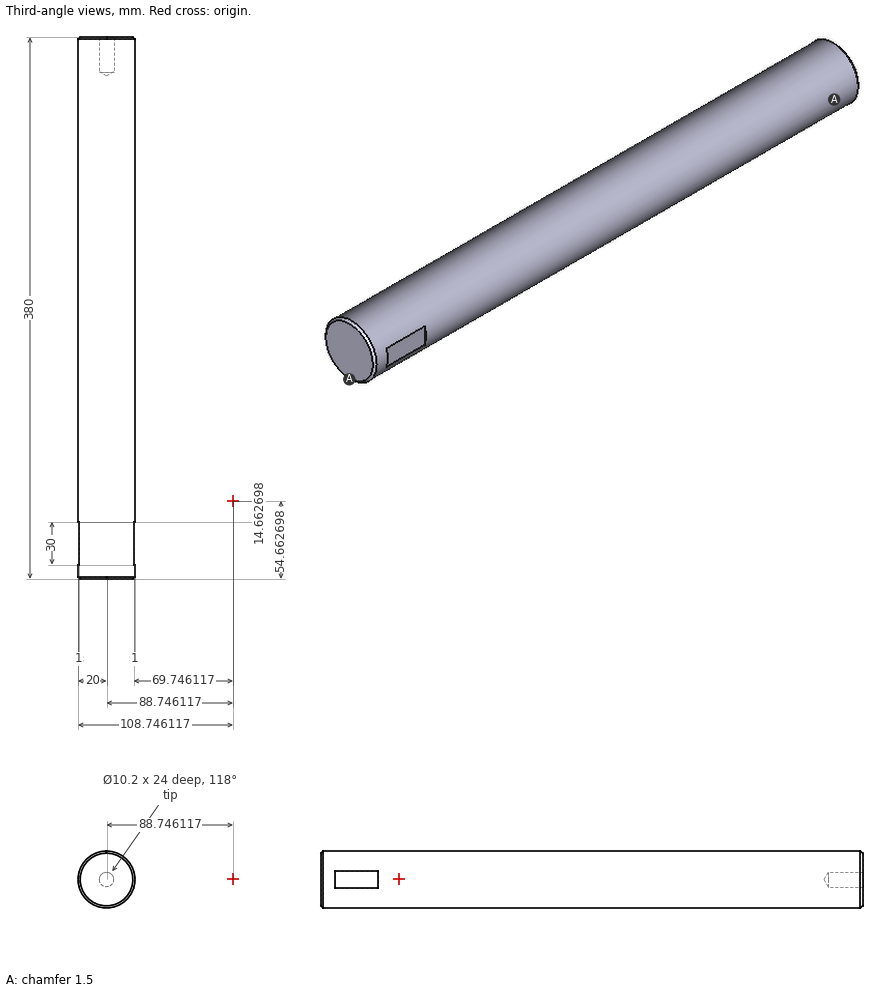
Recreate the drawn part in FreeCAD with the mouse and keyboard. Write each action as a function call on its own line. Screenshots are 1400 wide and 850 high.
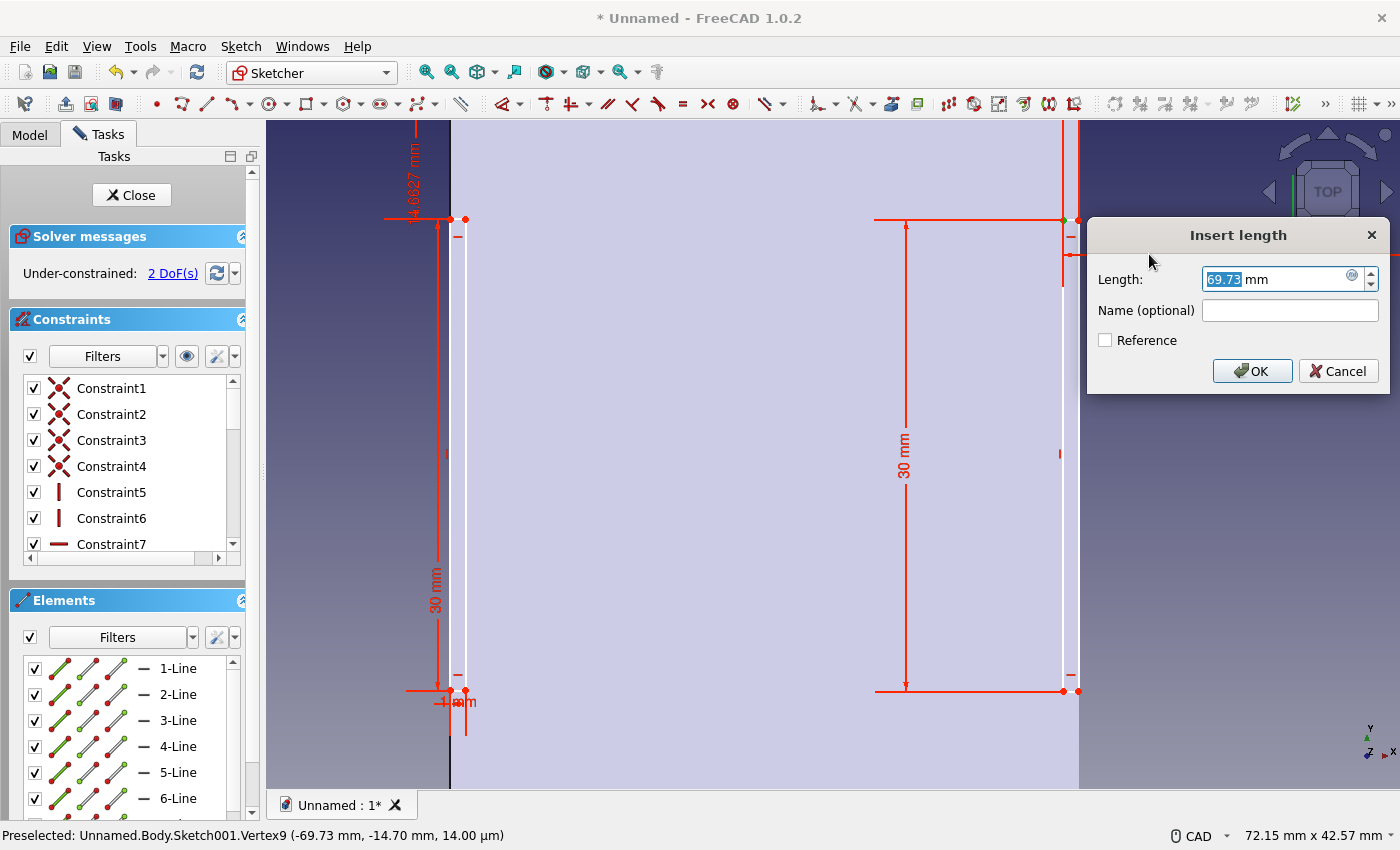
text(69.746117)
key(Return)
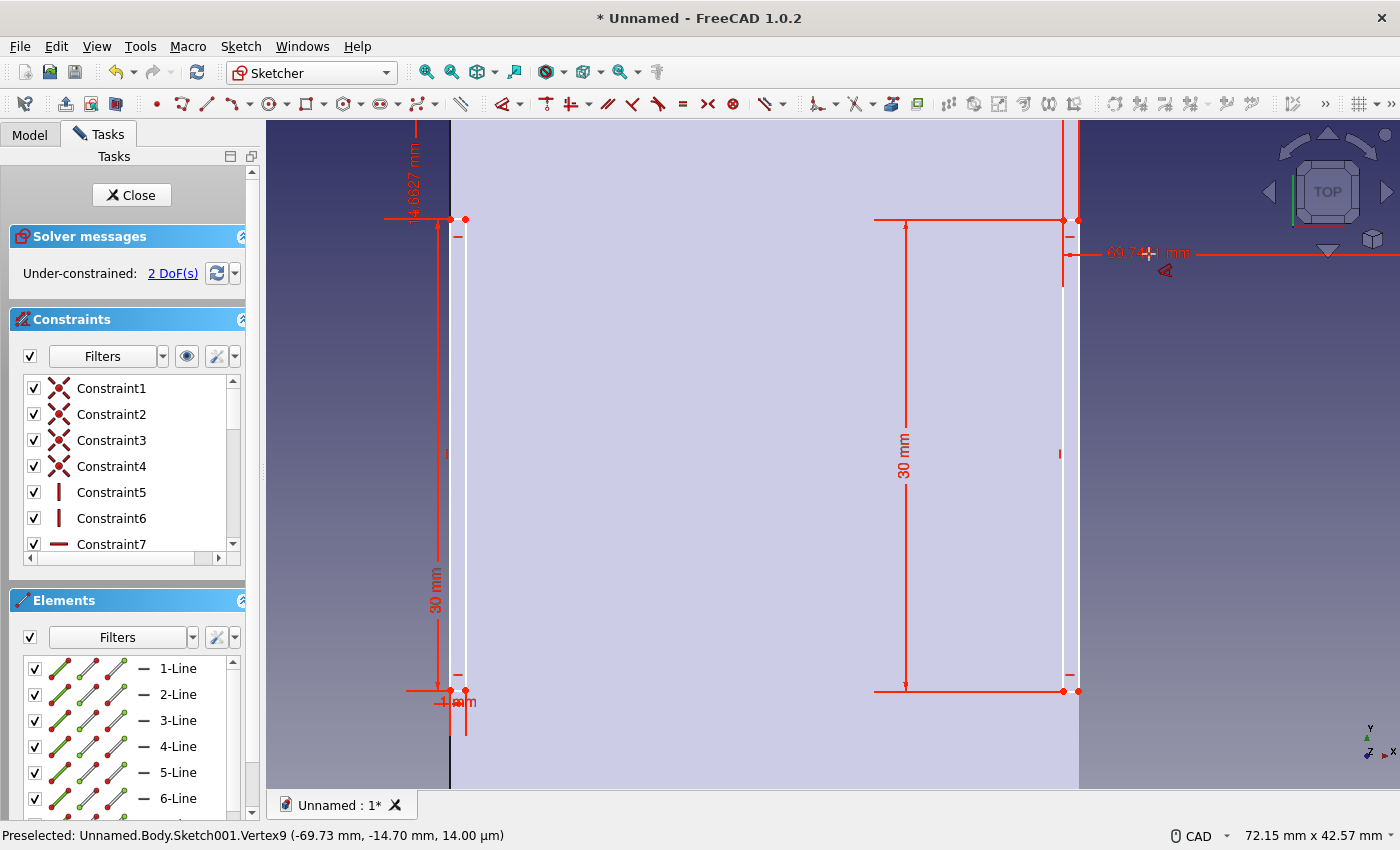
click(1063, 220)
click(1029, 184)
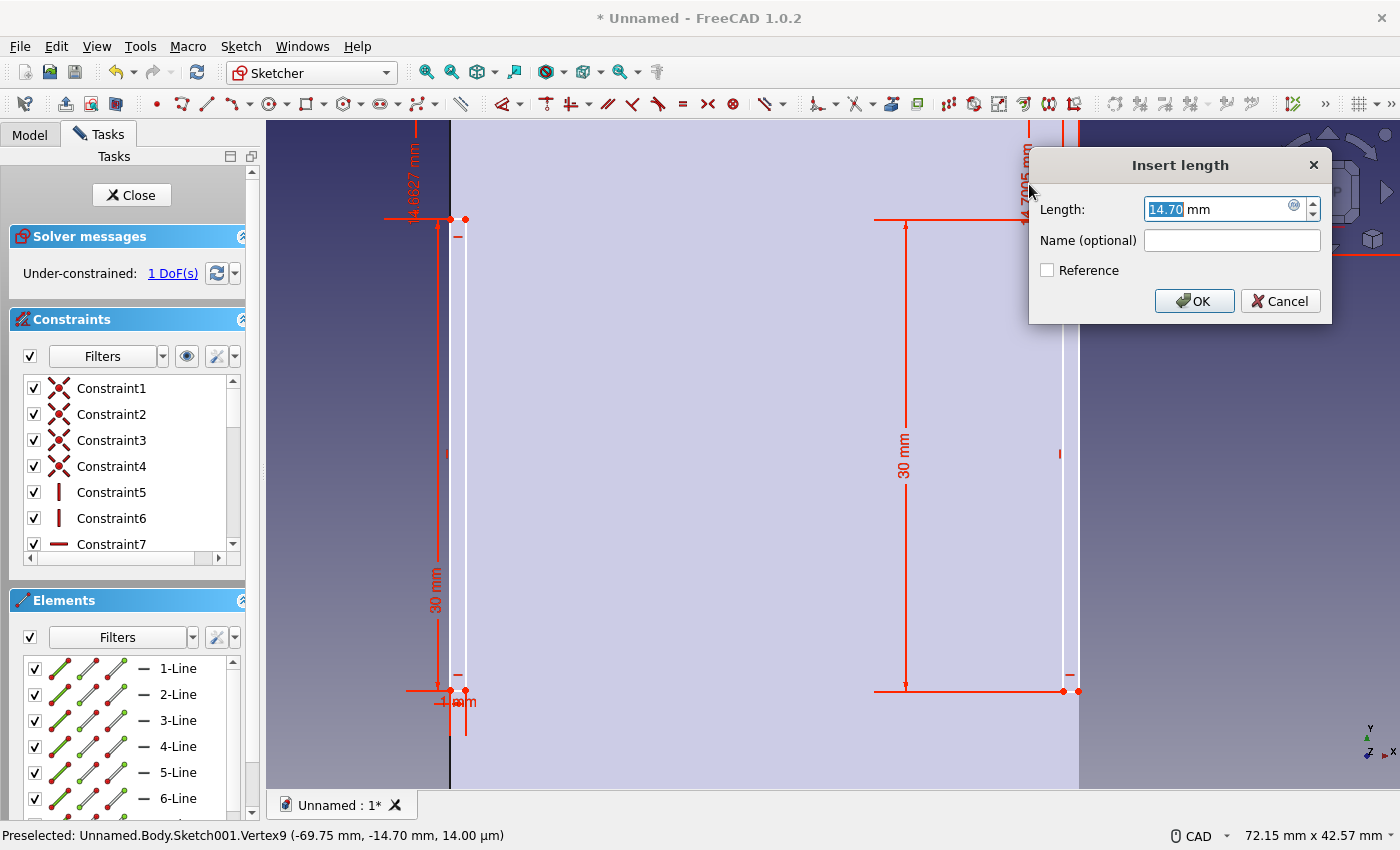
text(14.662698)
key(Return)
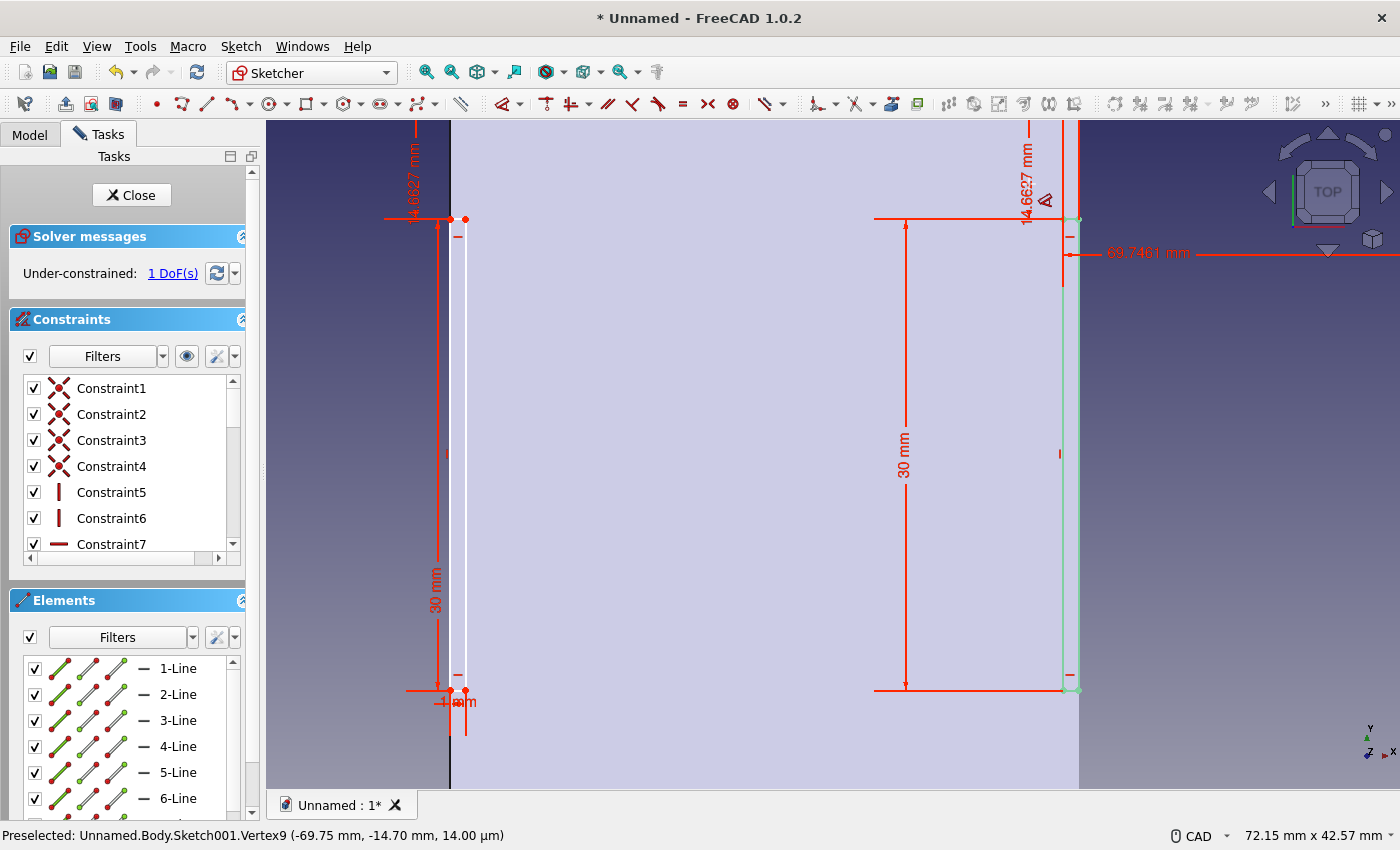
click(450, 219)
click(843, 253)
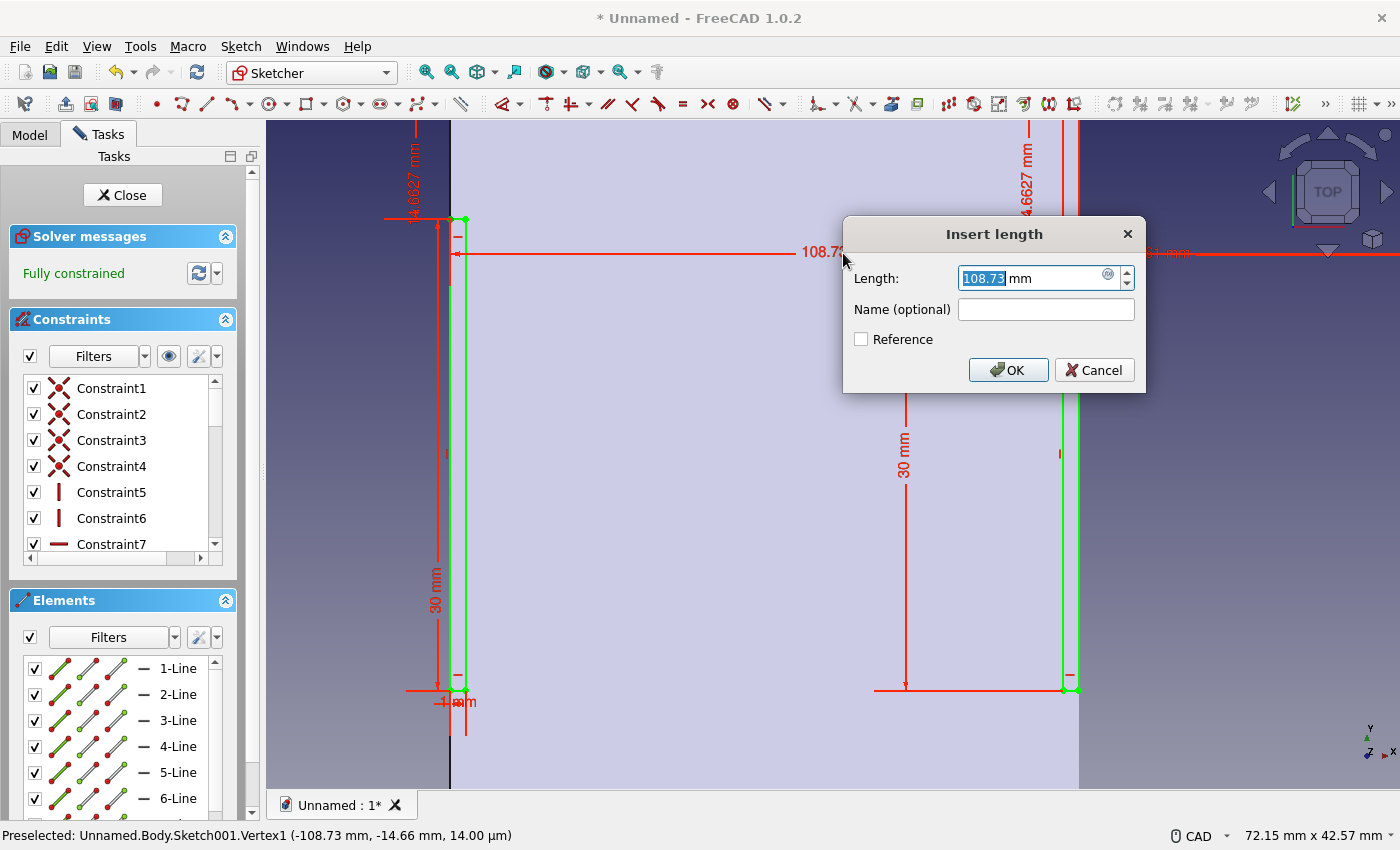
text(108.746117)
key(Return)
key(Escape)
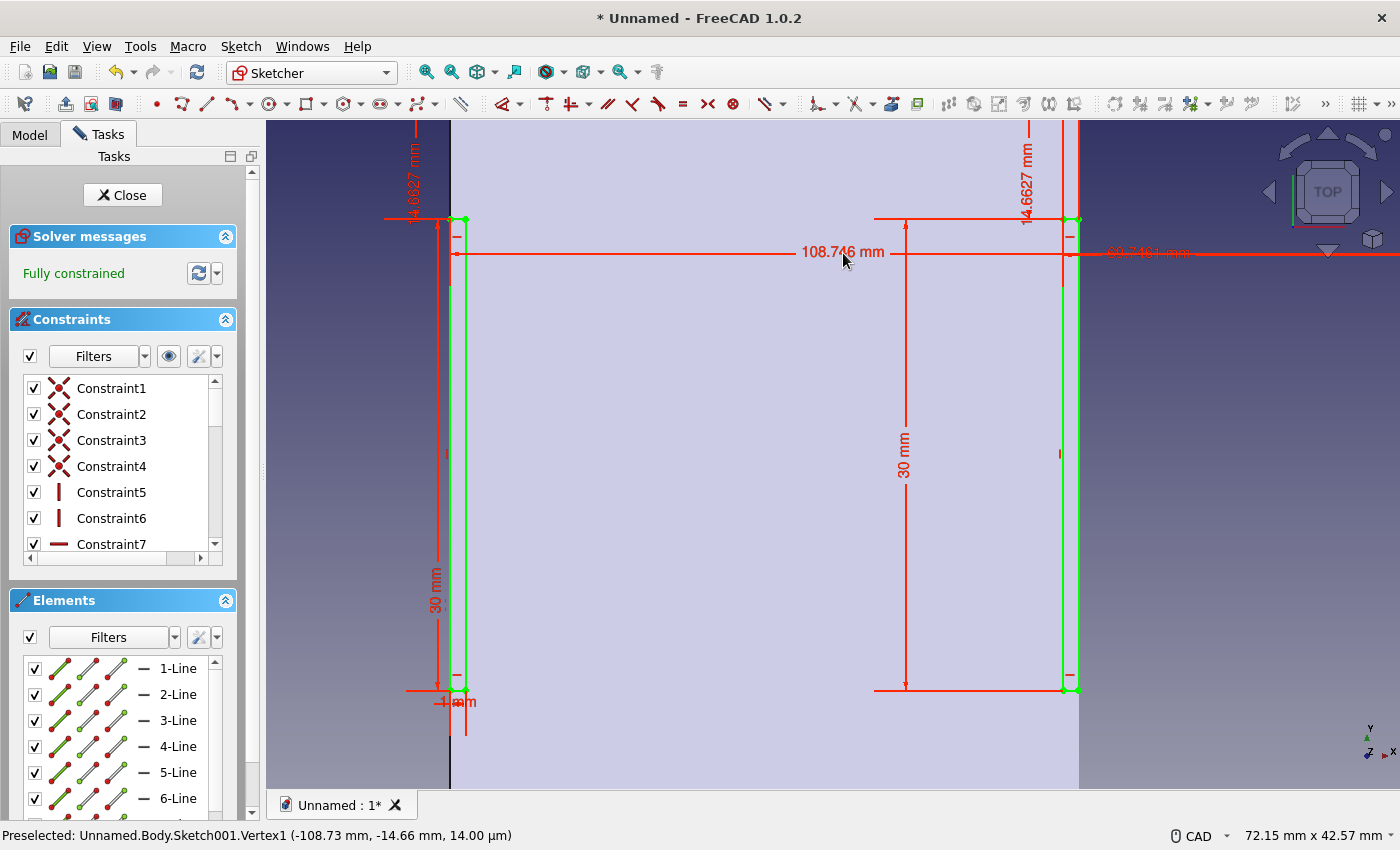
click(123, 195)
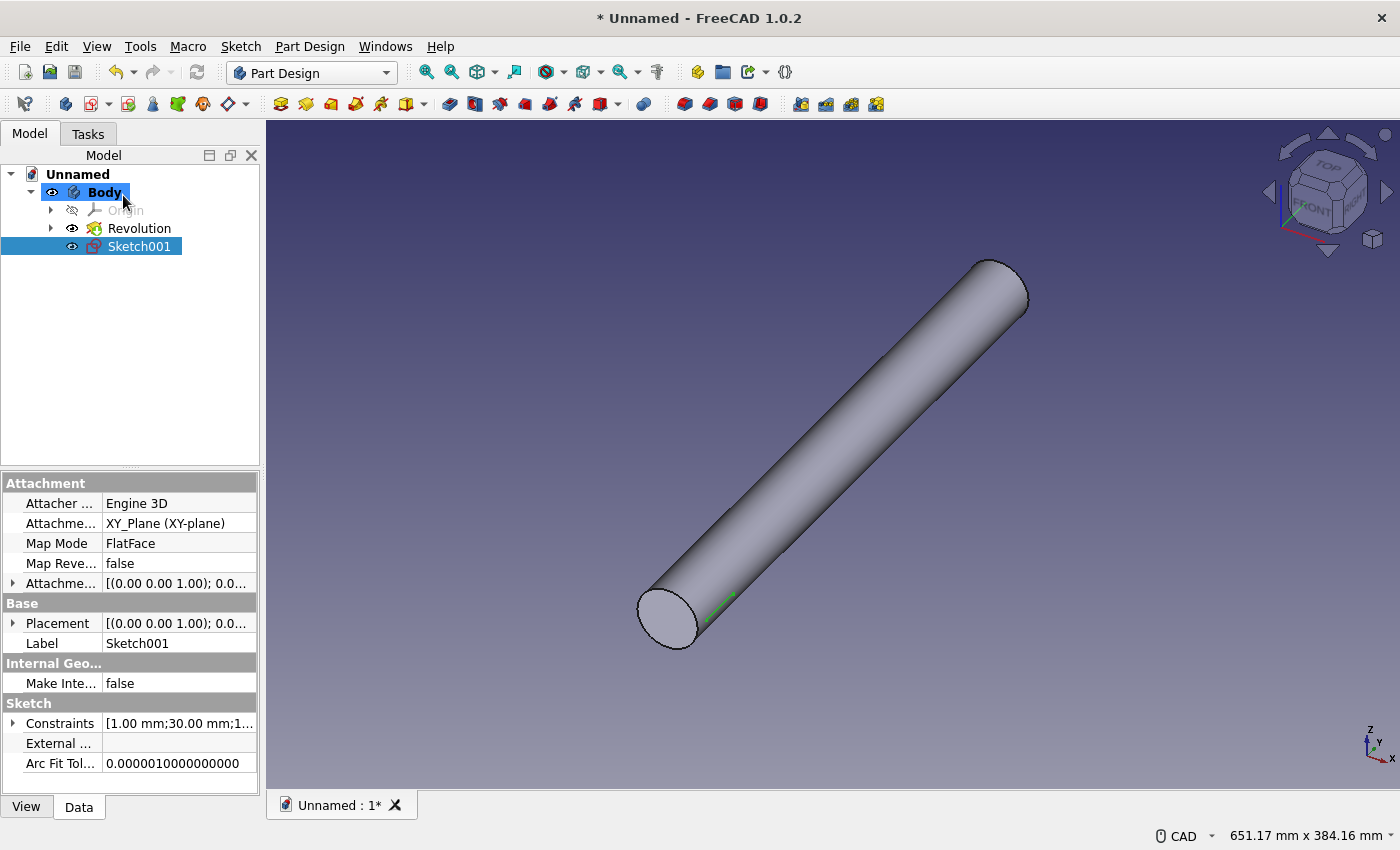
click(450, 104)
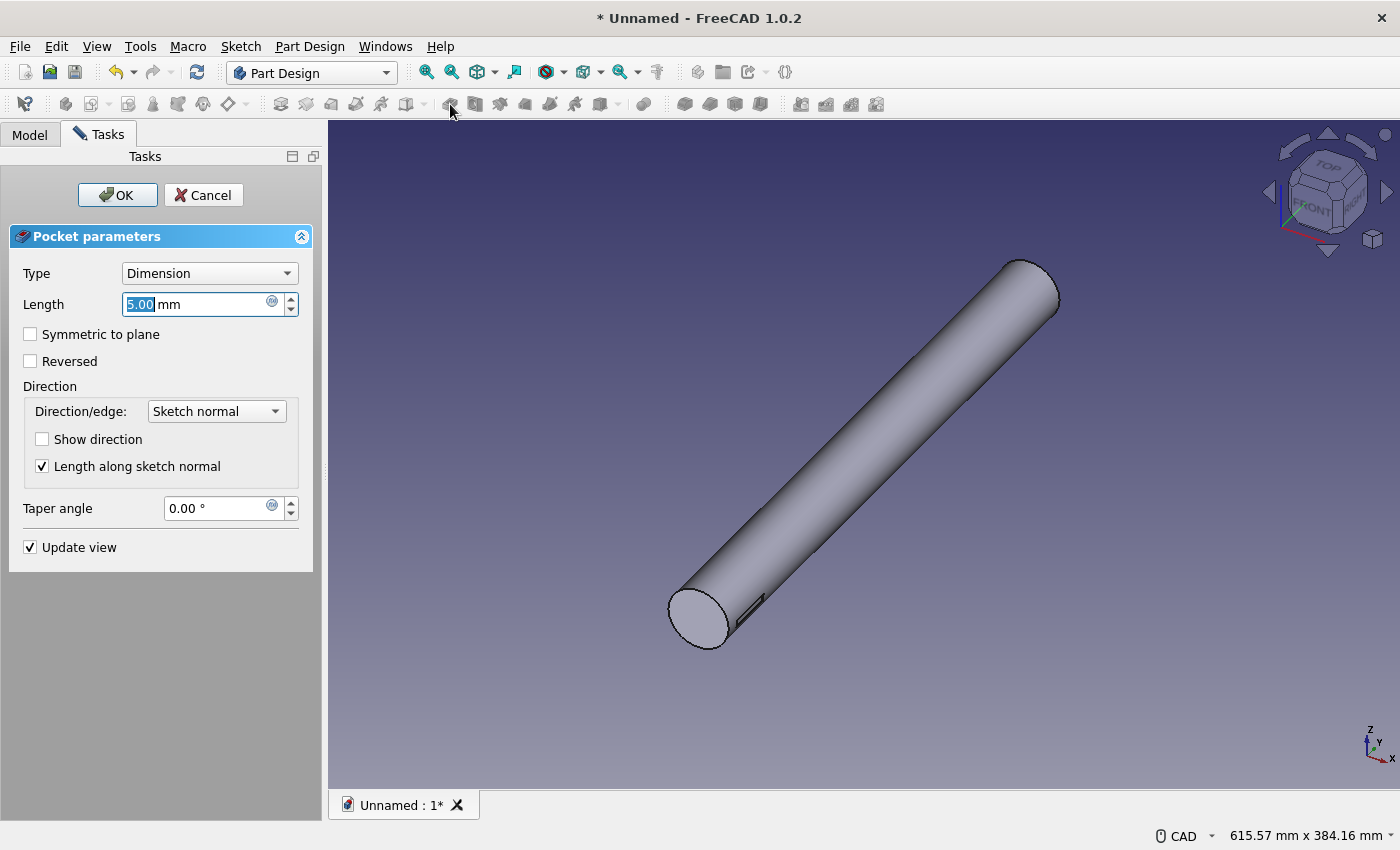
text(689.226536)
key(Tab)